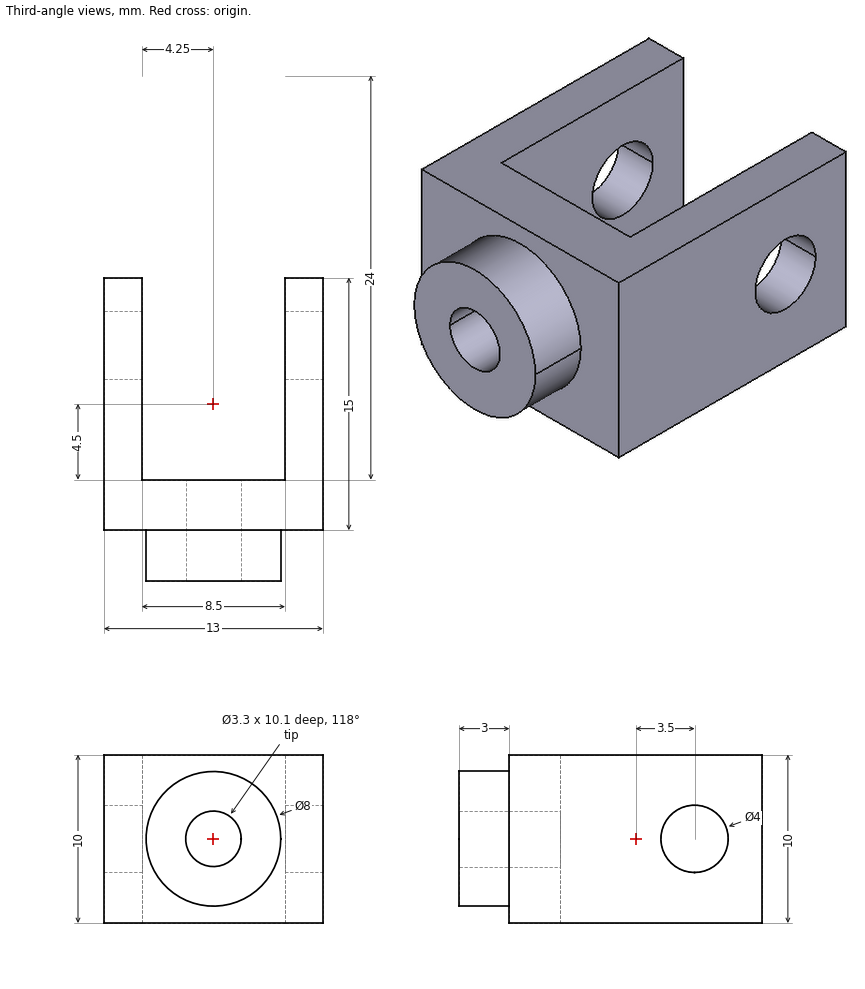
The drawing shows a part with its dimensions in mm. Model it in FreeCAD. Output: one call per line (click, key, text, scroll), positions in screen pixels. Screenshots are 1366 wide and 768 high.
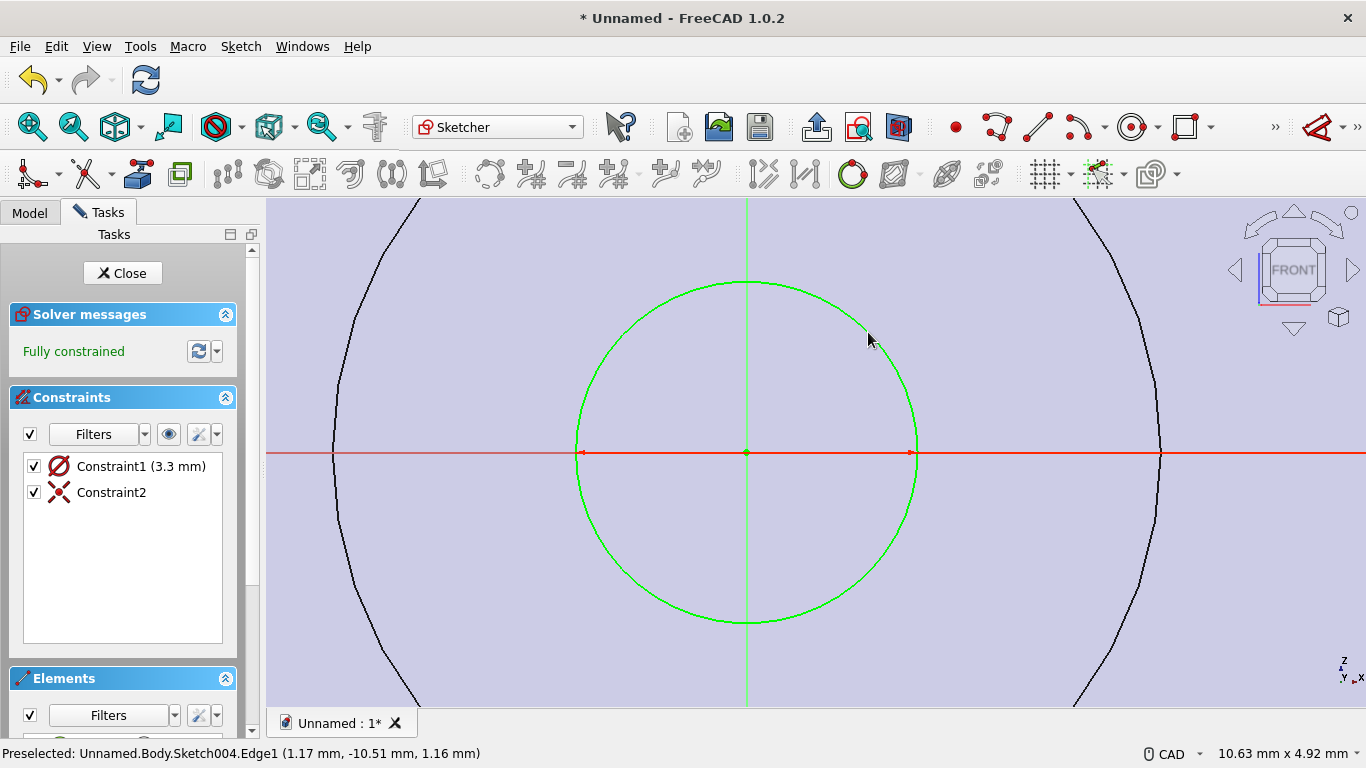
click(123, 273)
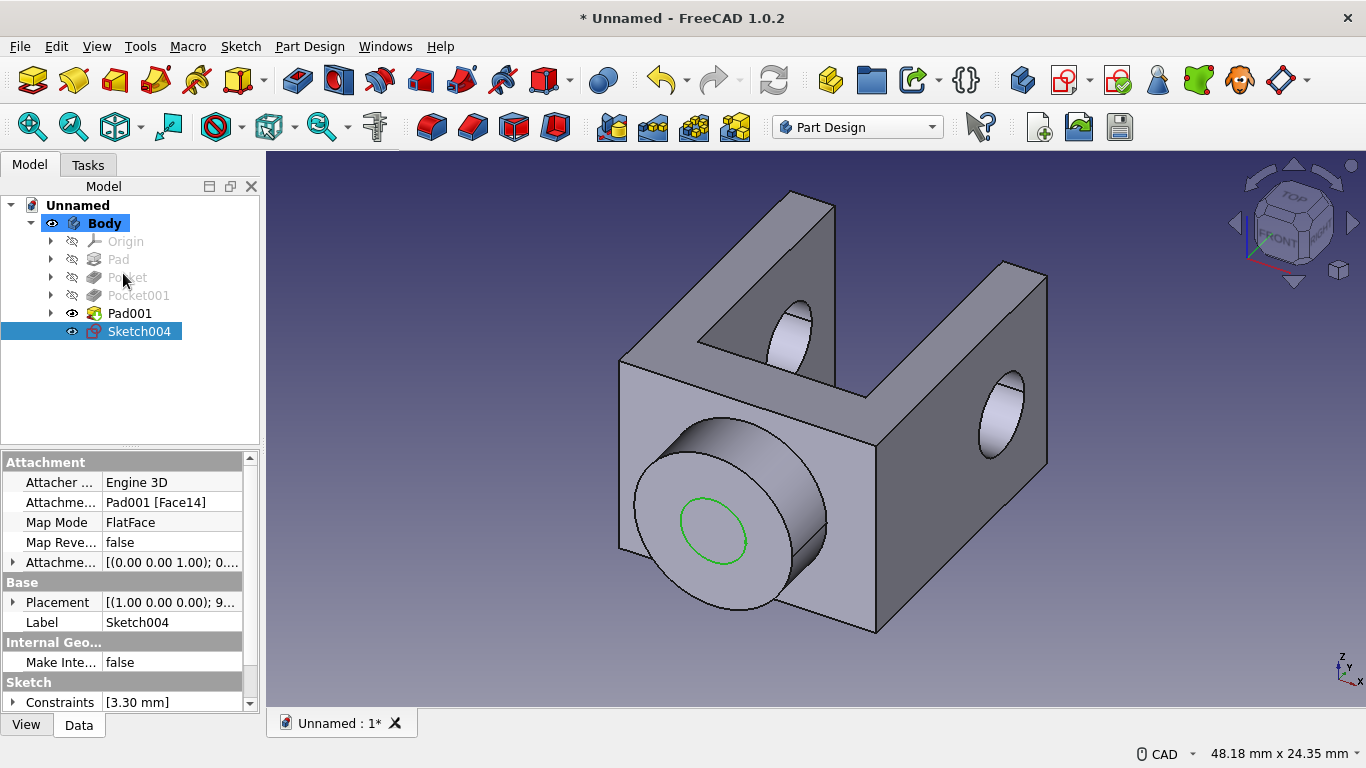
click(339, 80)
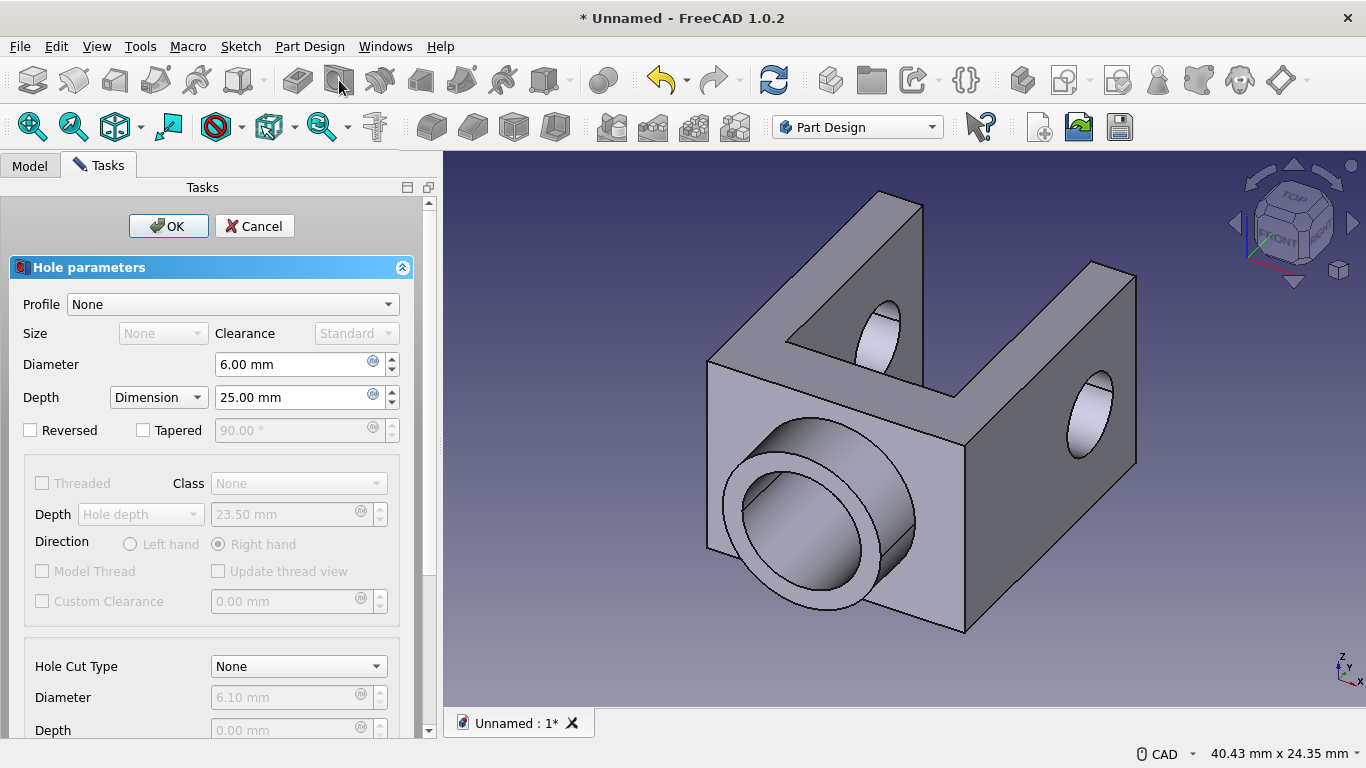
triple_click(300, 364)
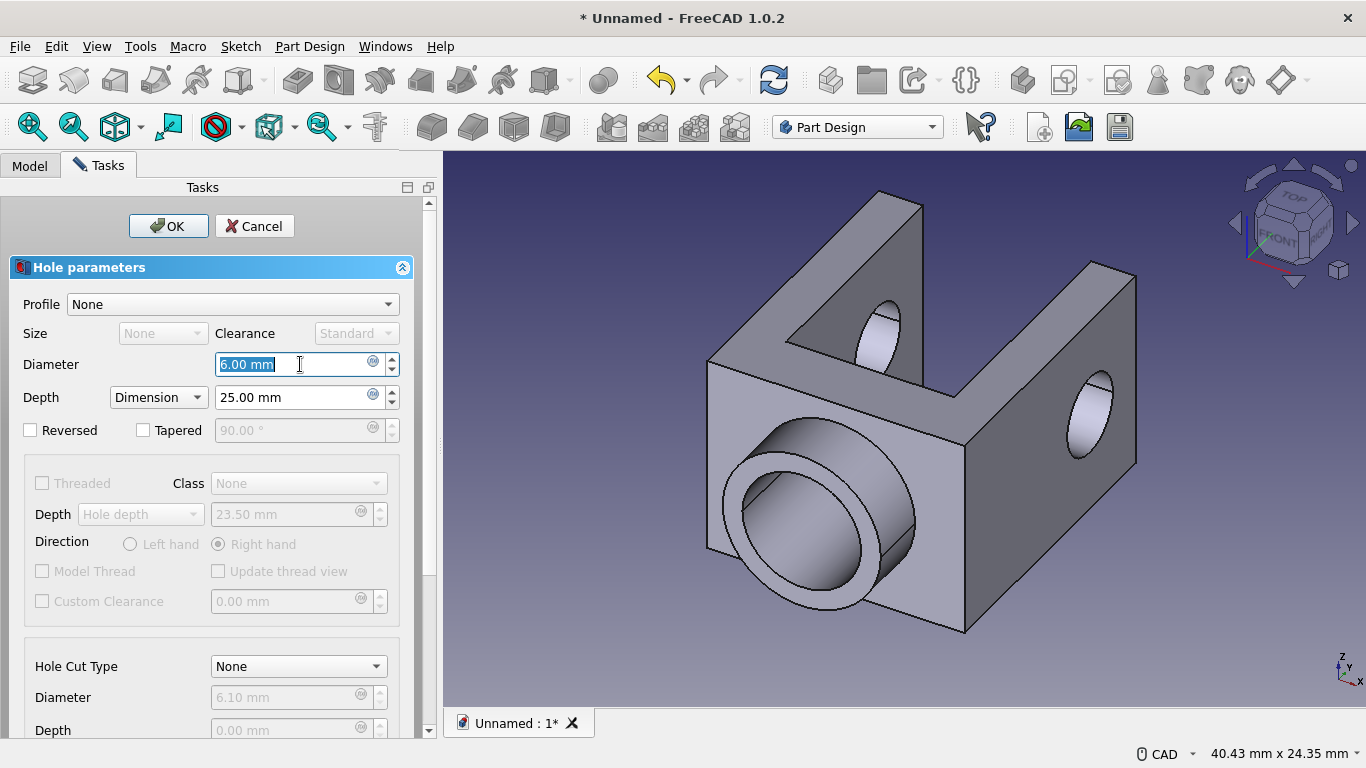
text(3.3)
key(Tab)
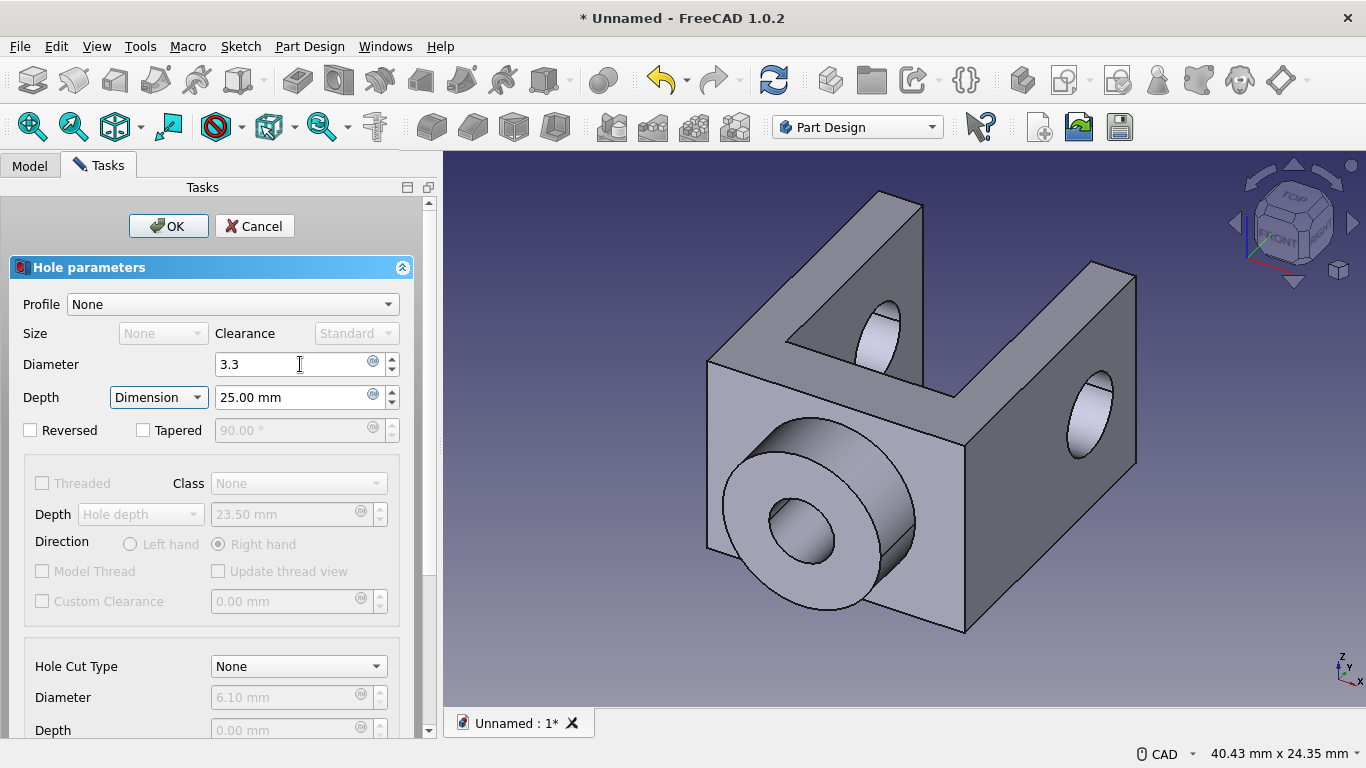
triple_click(300, 398)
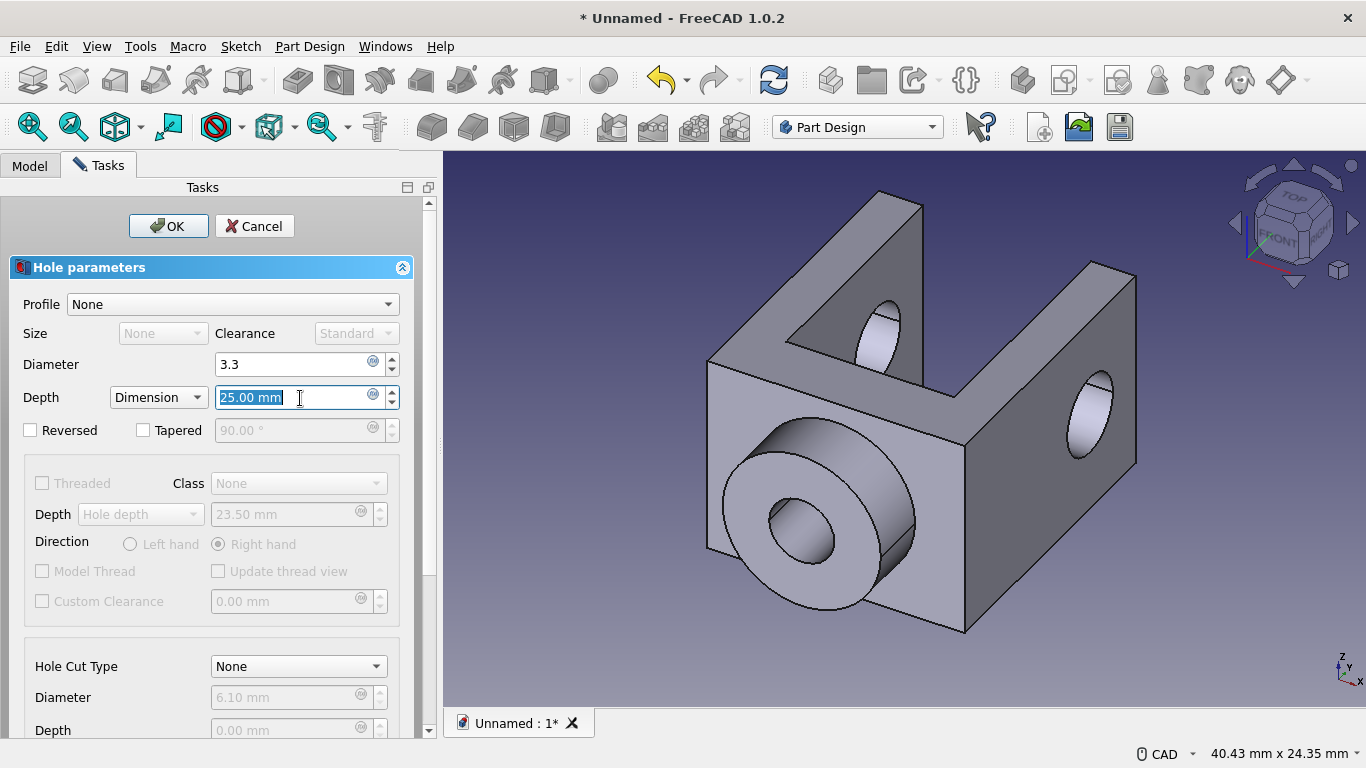
text(10.1)
key(Tab)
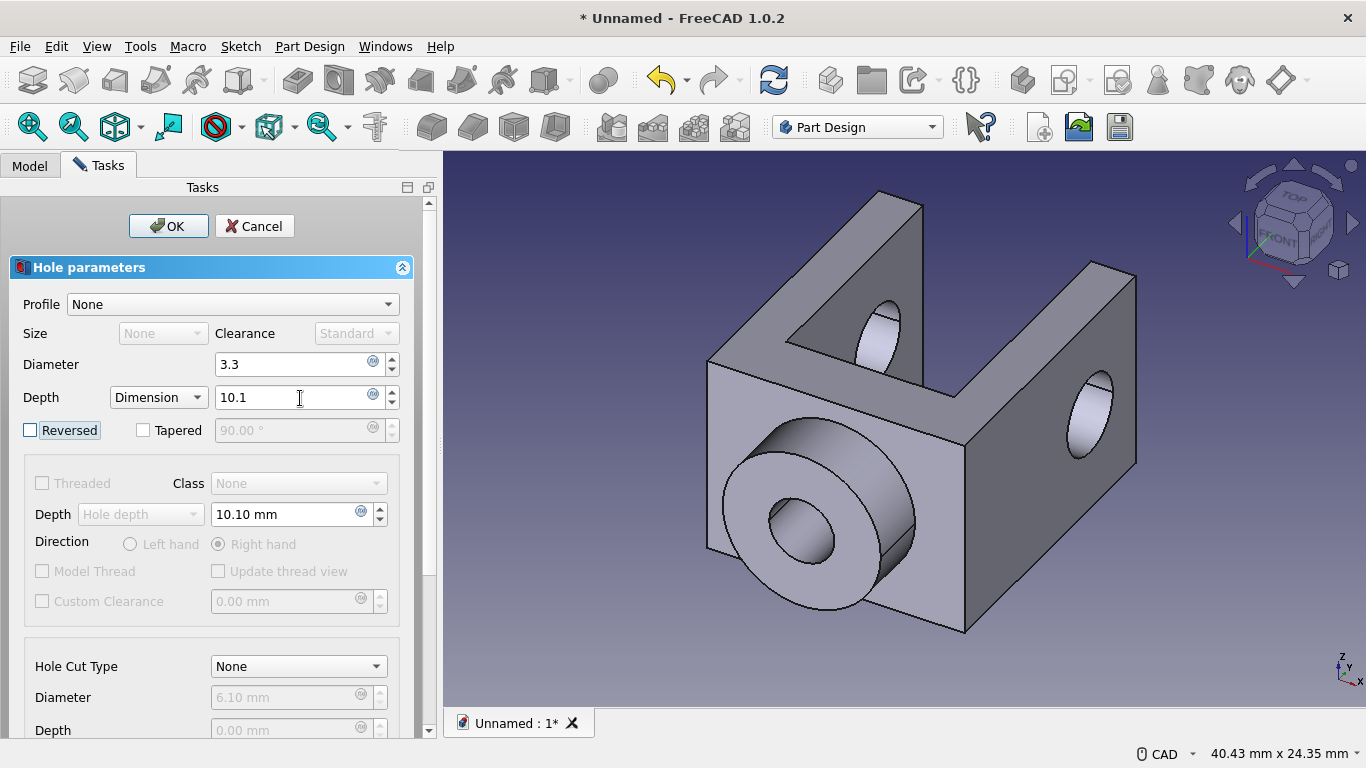
click(169, 226)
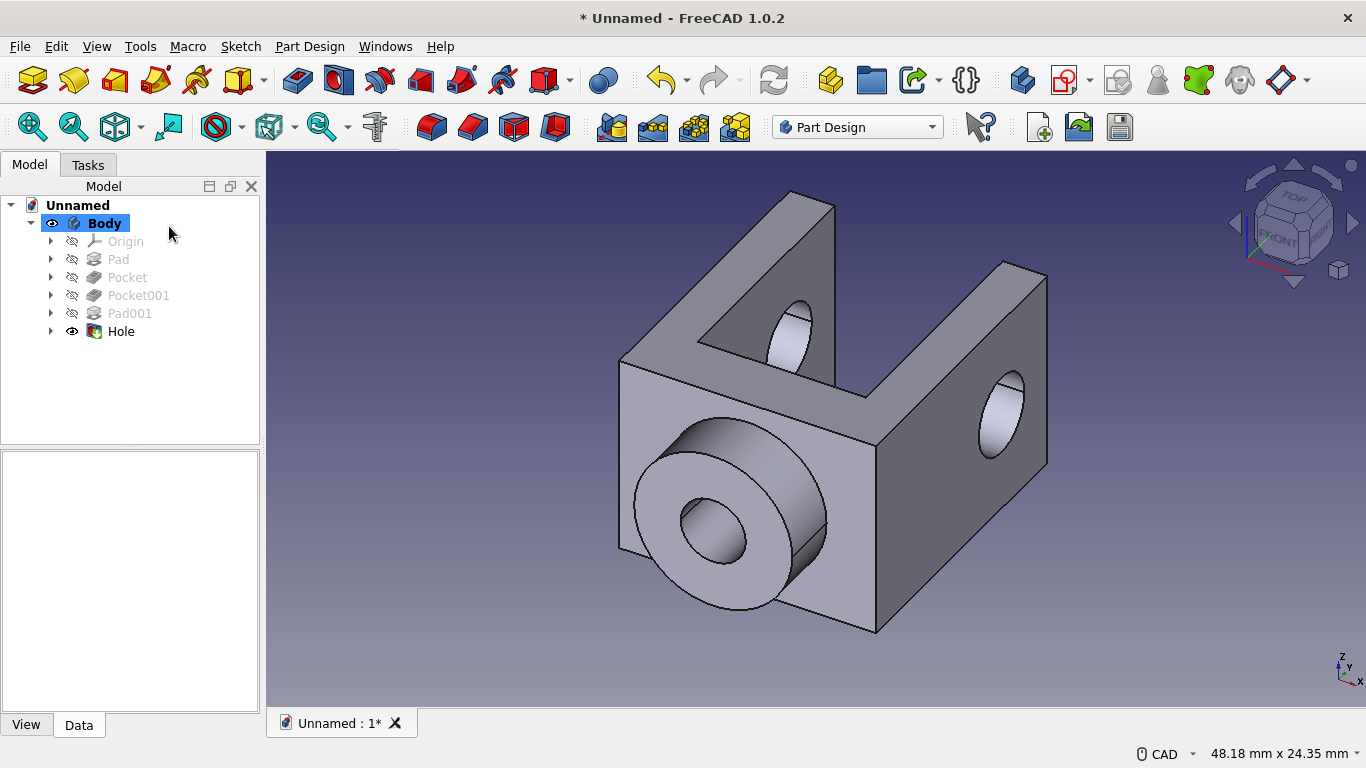
key(0)